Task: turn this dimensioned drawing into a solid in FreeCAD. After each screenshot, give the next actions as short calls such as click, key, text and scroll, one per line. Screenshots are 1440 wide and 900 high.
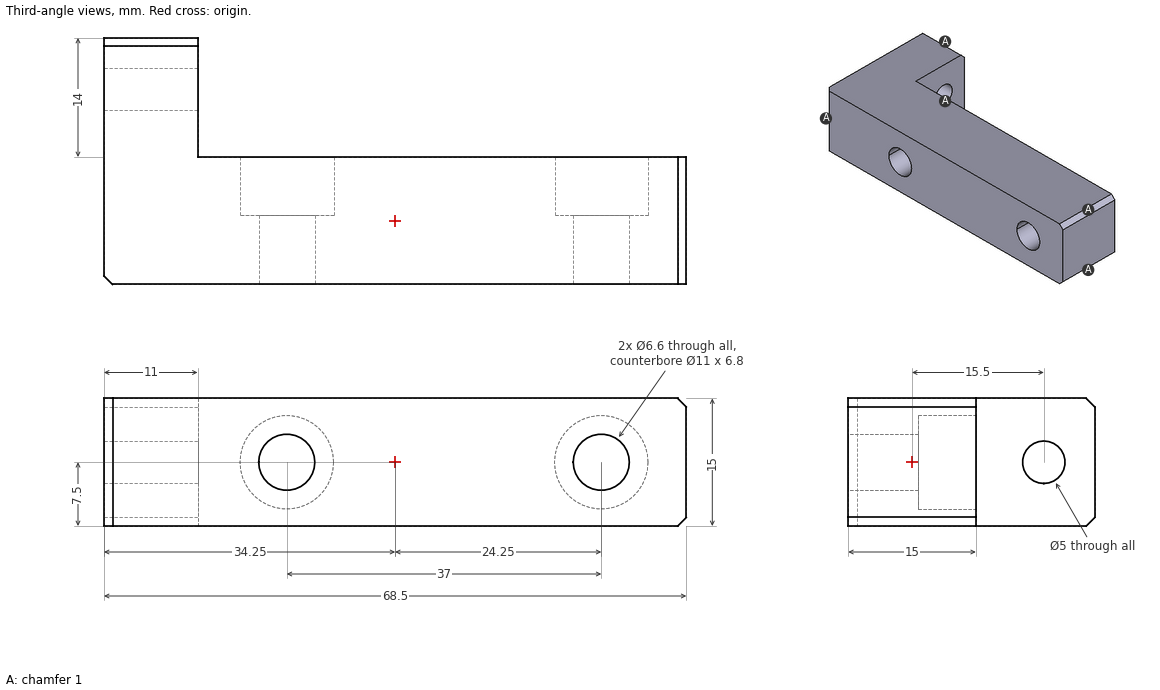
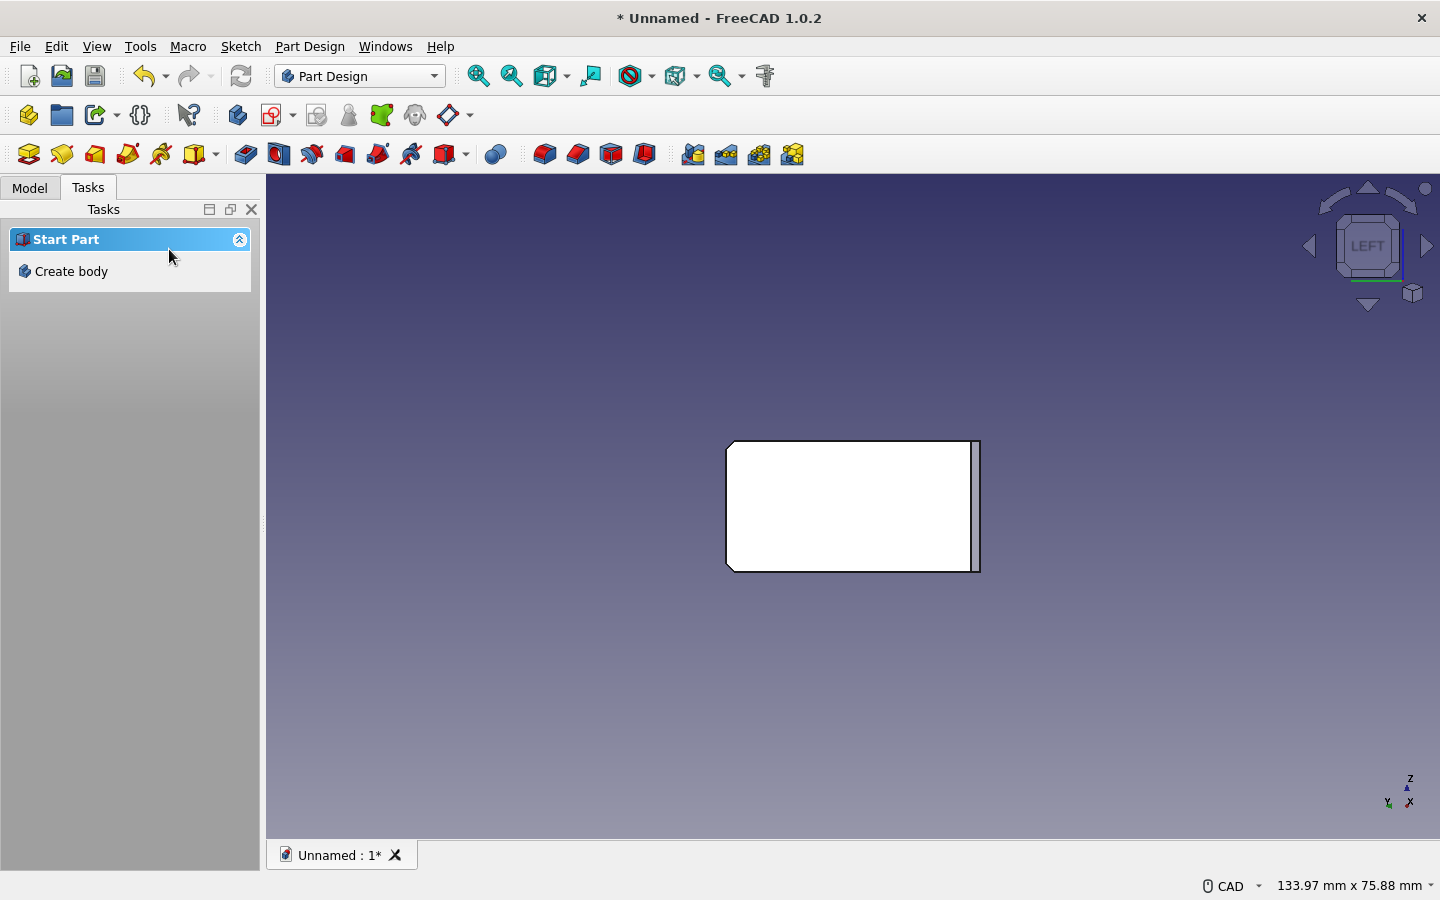
click(479, 76)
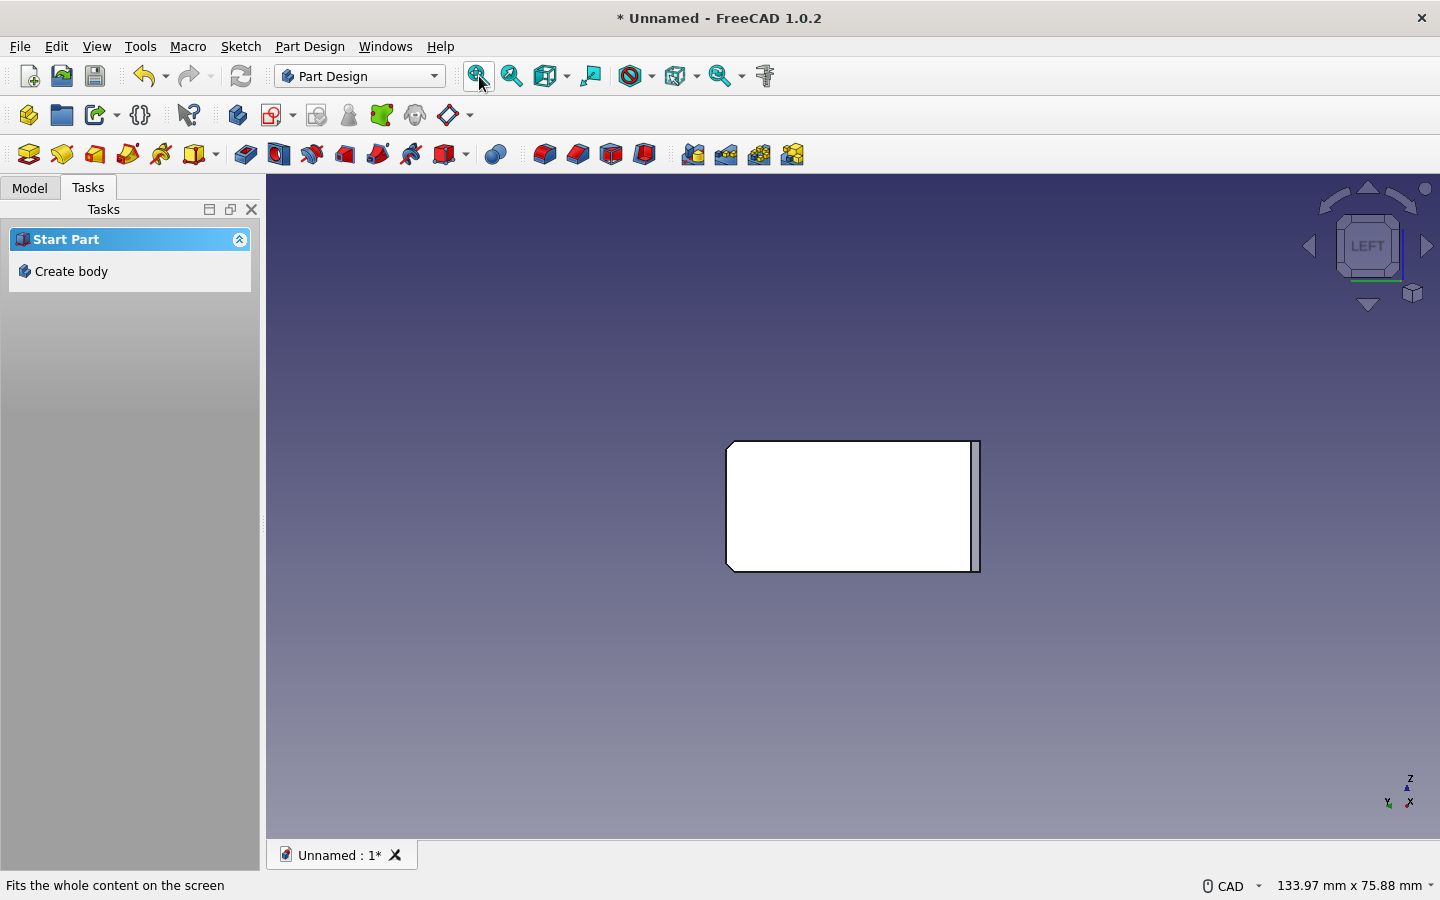
click(849, 505)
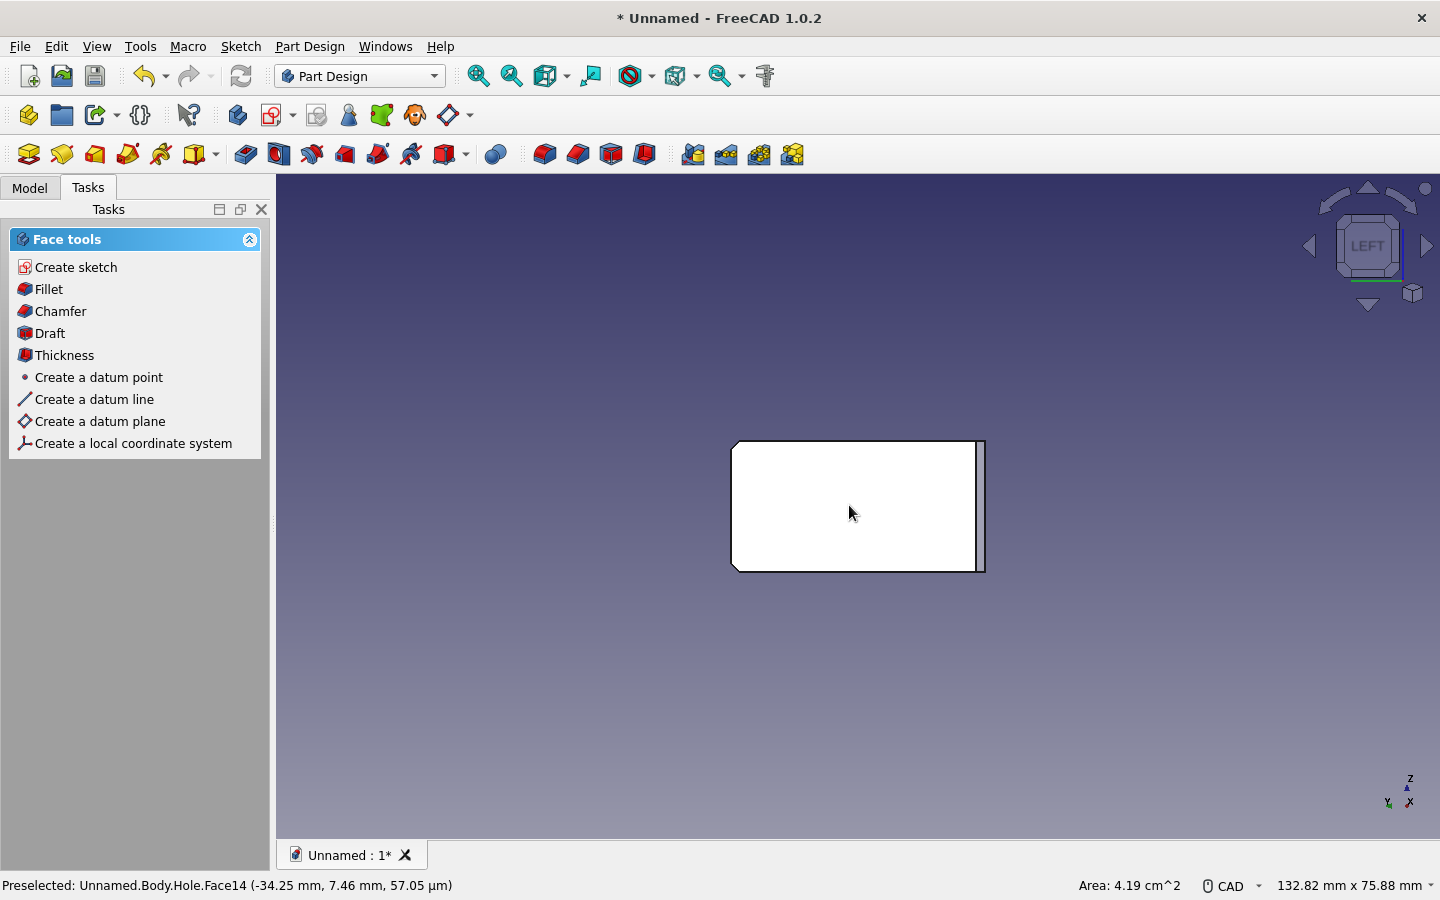
click(270, 116)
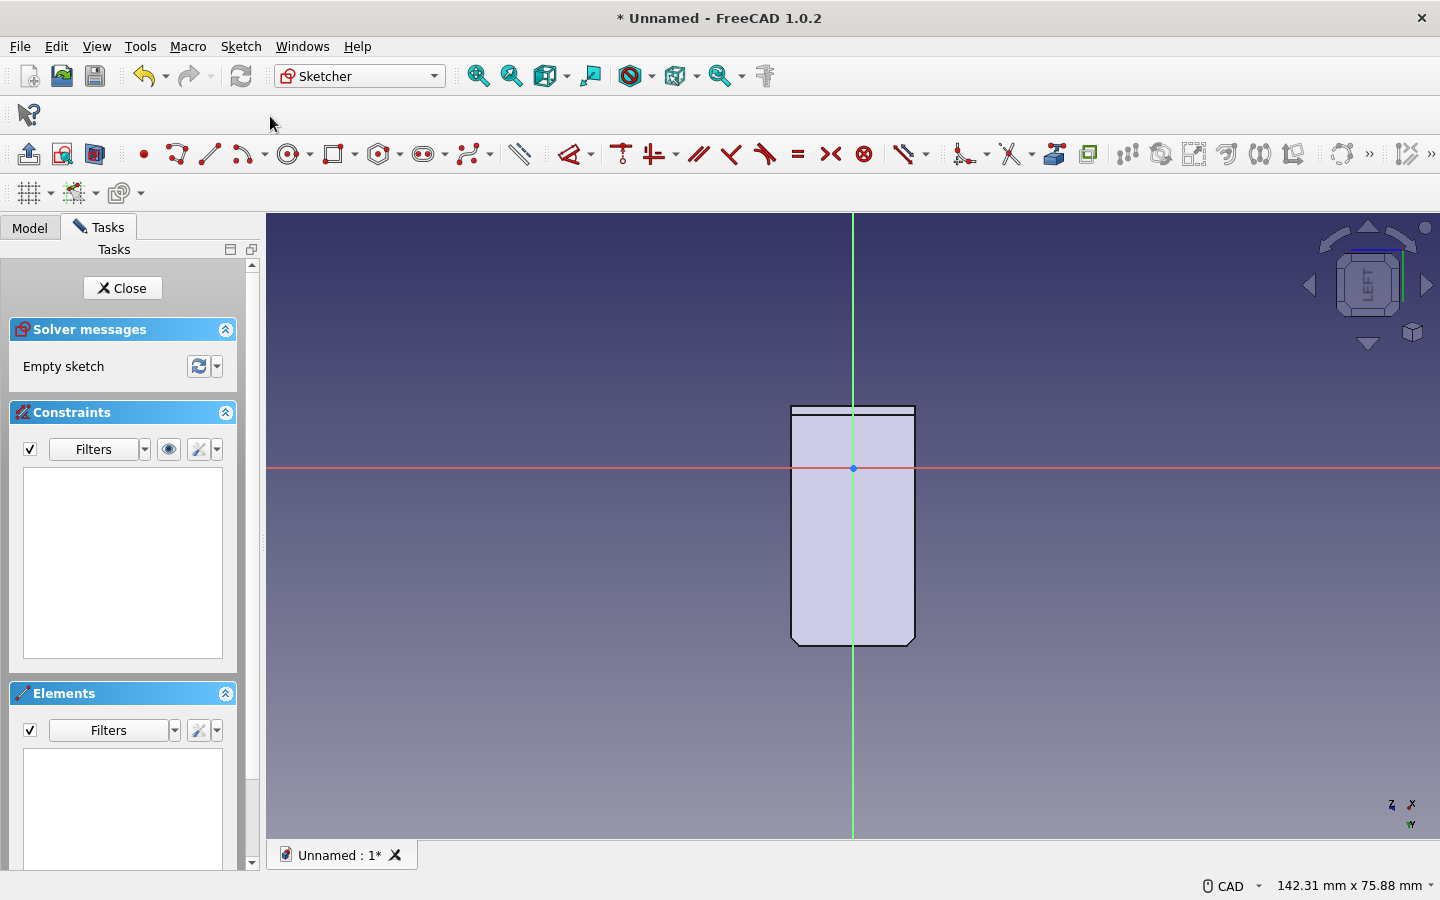
scroll(862, 605, up, 11)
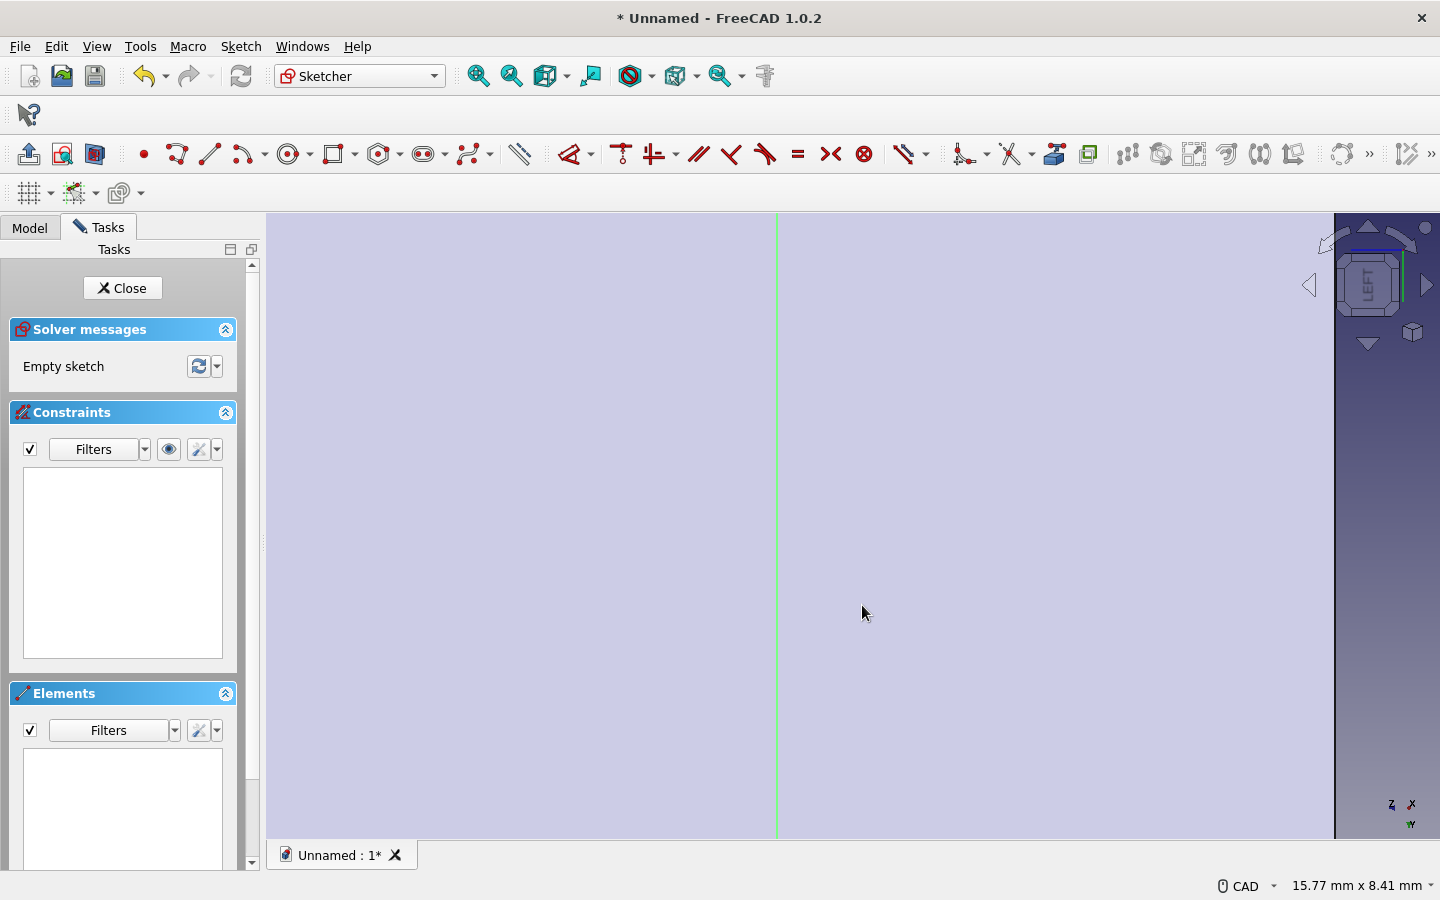
click(288, 154)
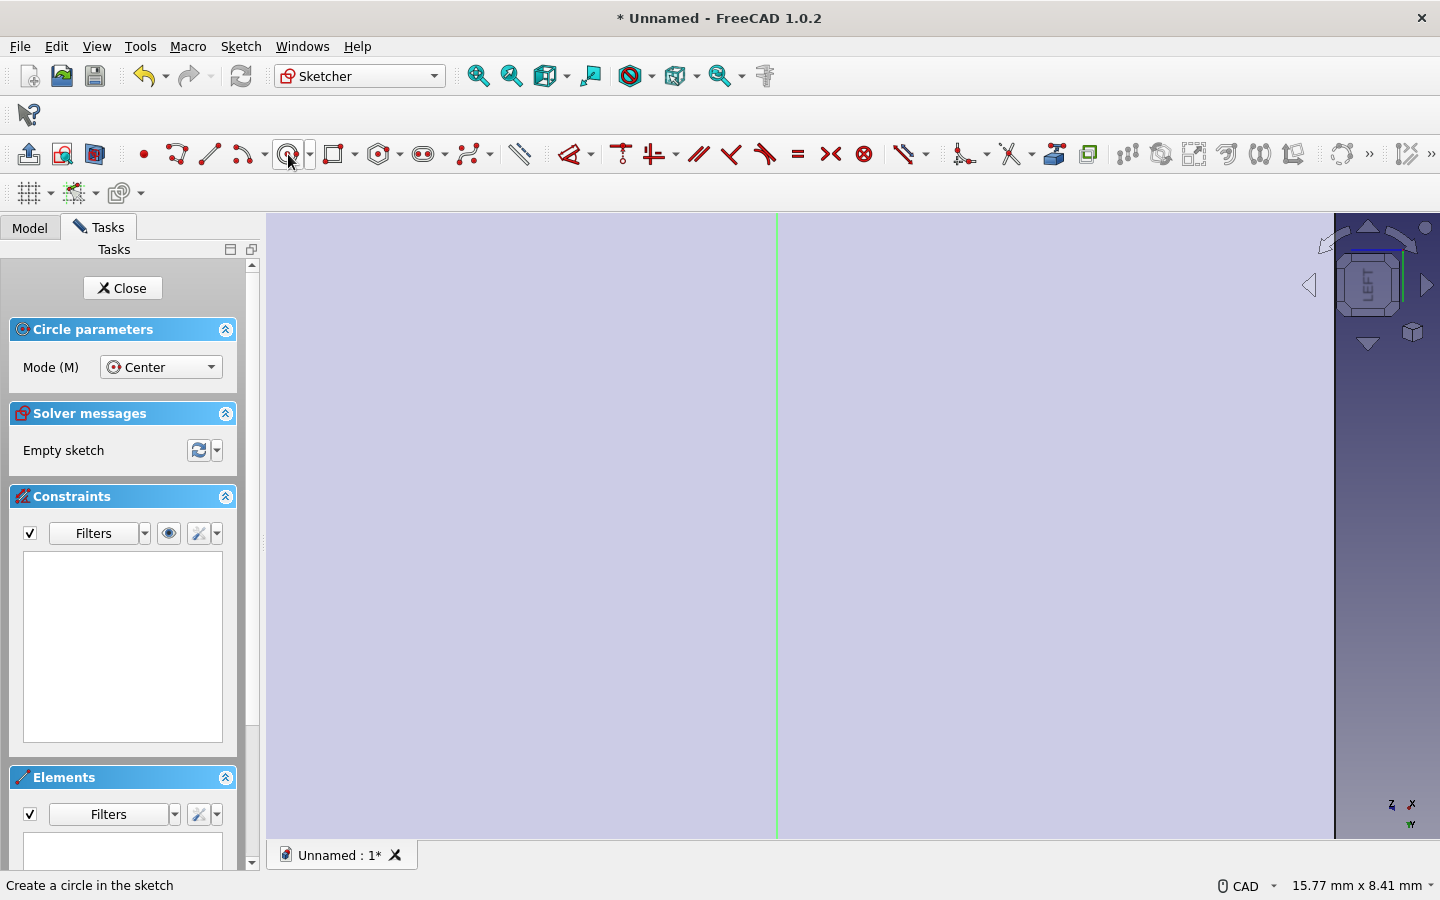
click(777, 520)
move(908, 388)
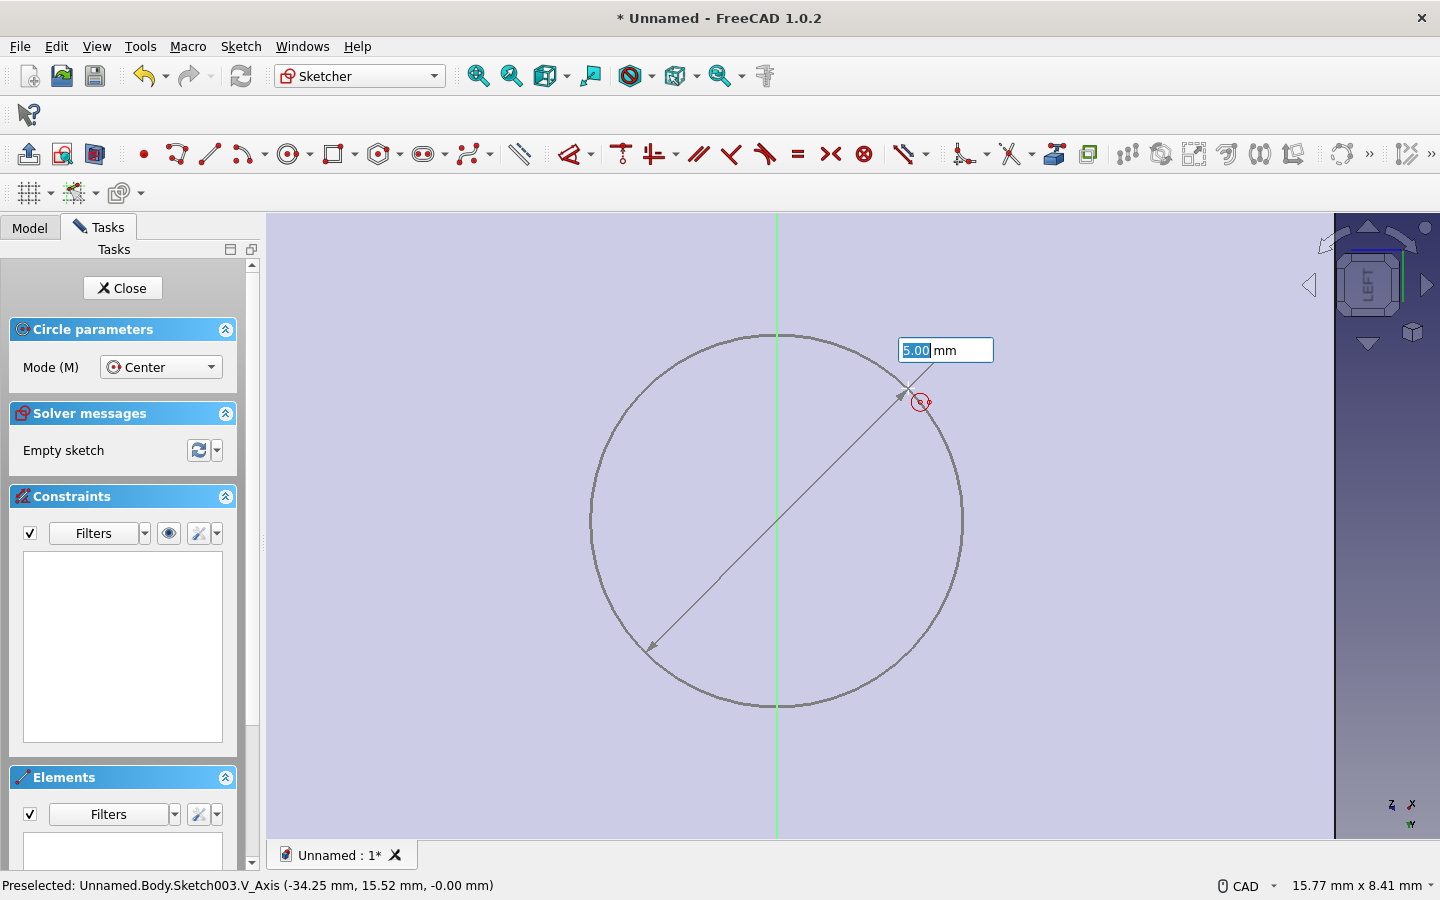
text(5)
key(Return)
key(Escape)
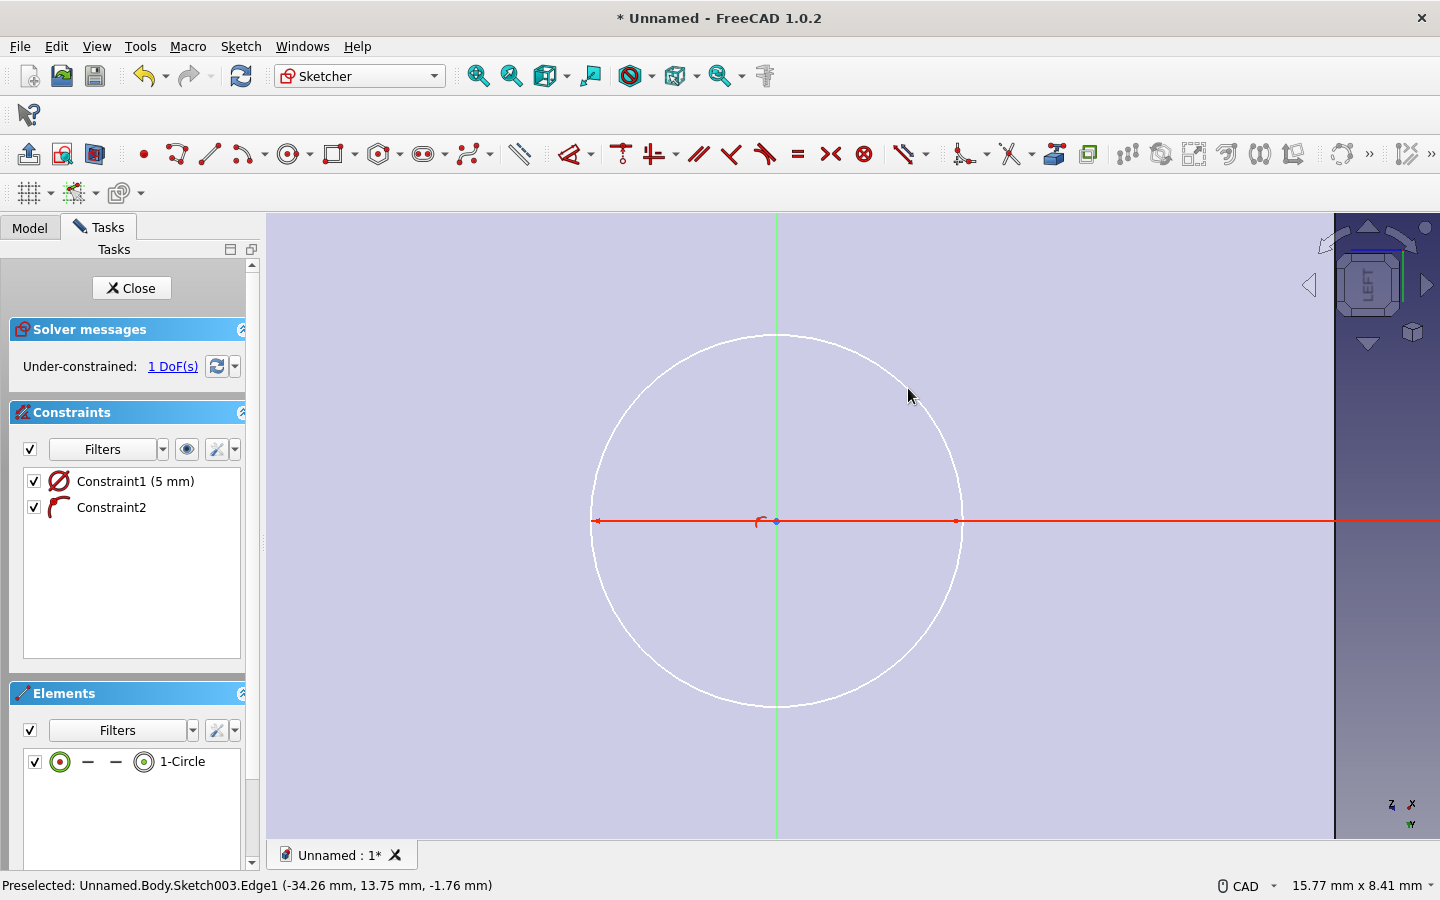
click(568, 154)